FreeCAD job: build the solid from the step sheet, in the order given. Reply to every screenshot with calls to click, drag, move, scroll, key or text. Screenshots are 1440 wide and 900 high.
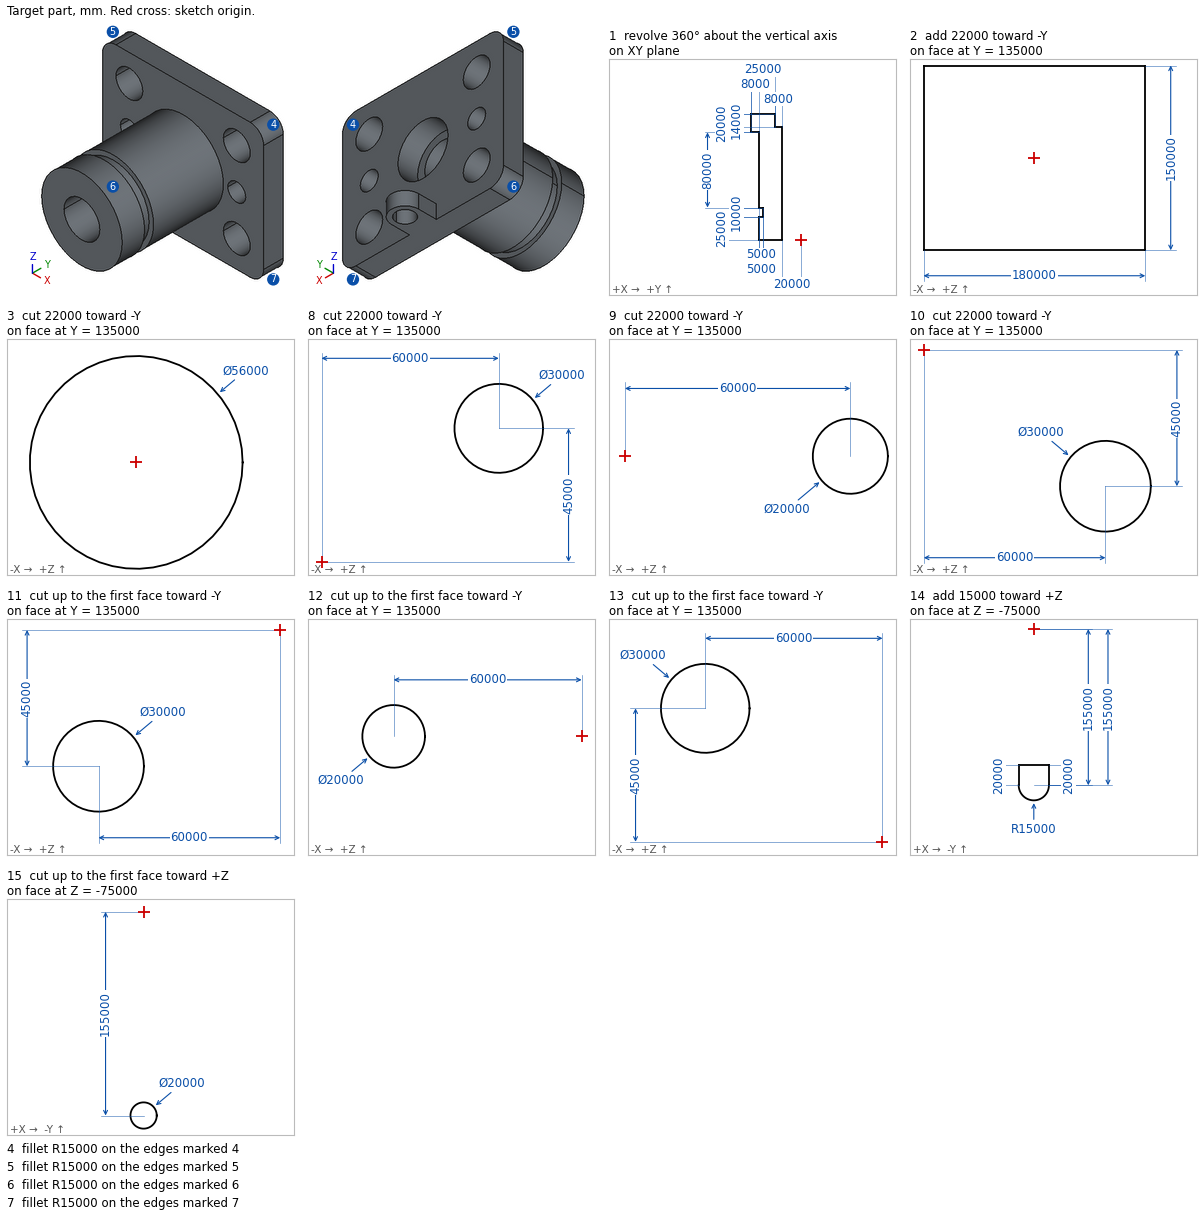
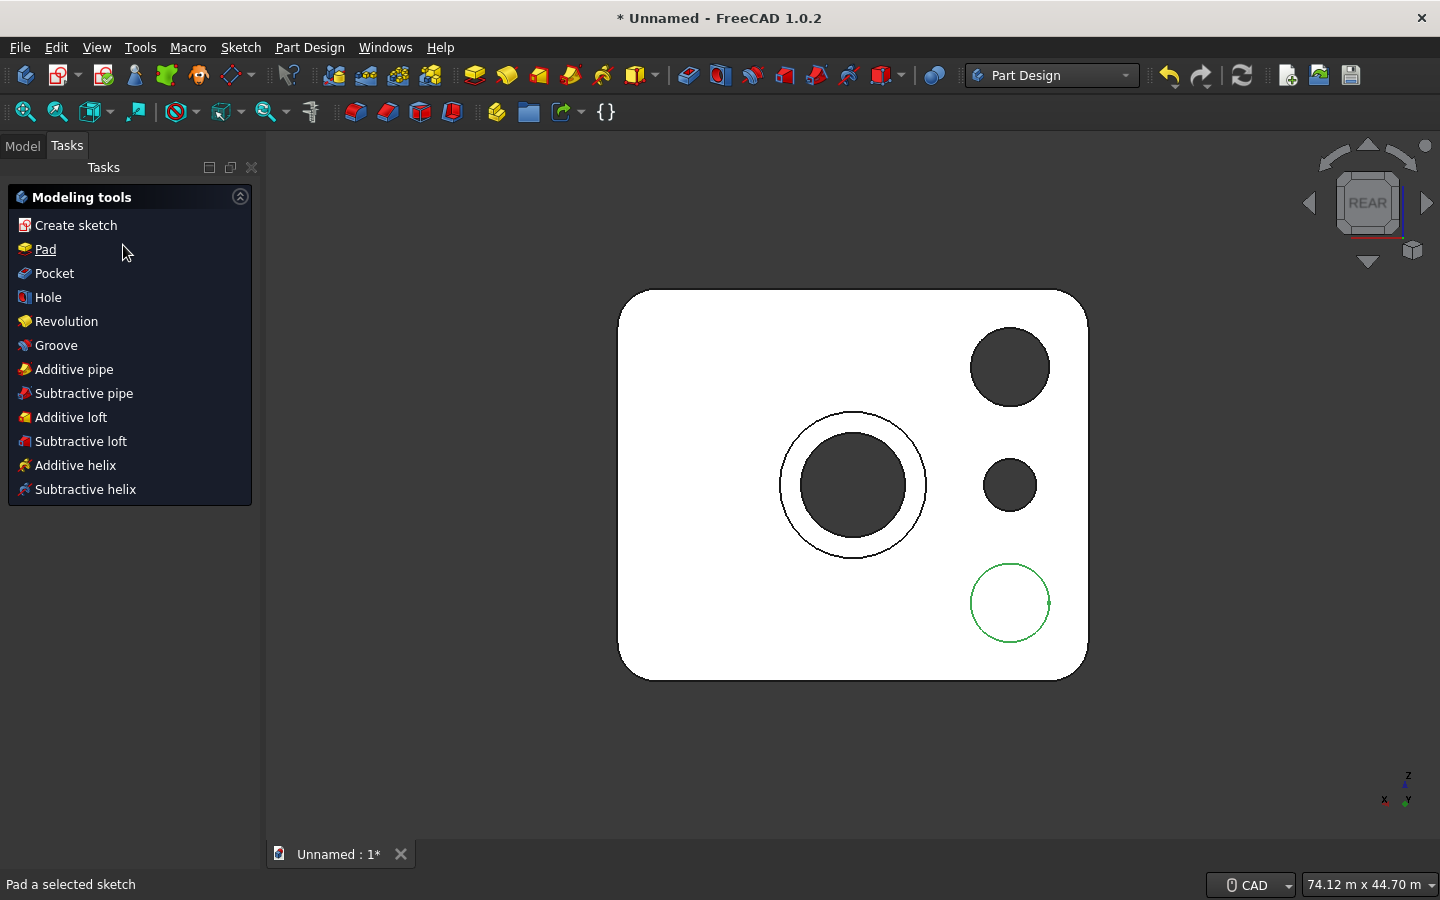
click(690, 76)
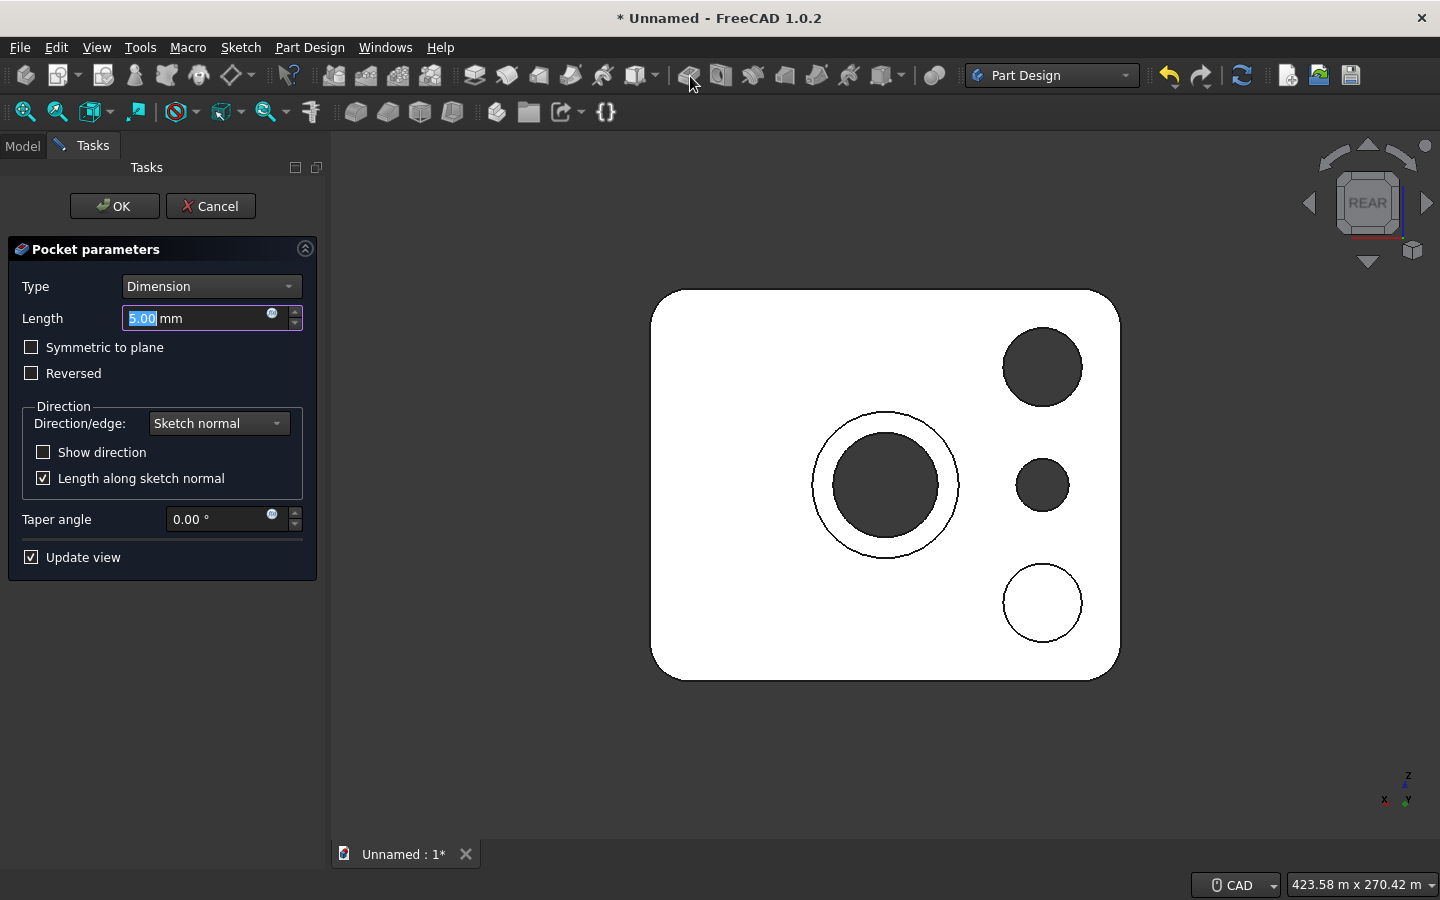
text(22000)
key(Tab)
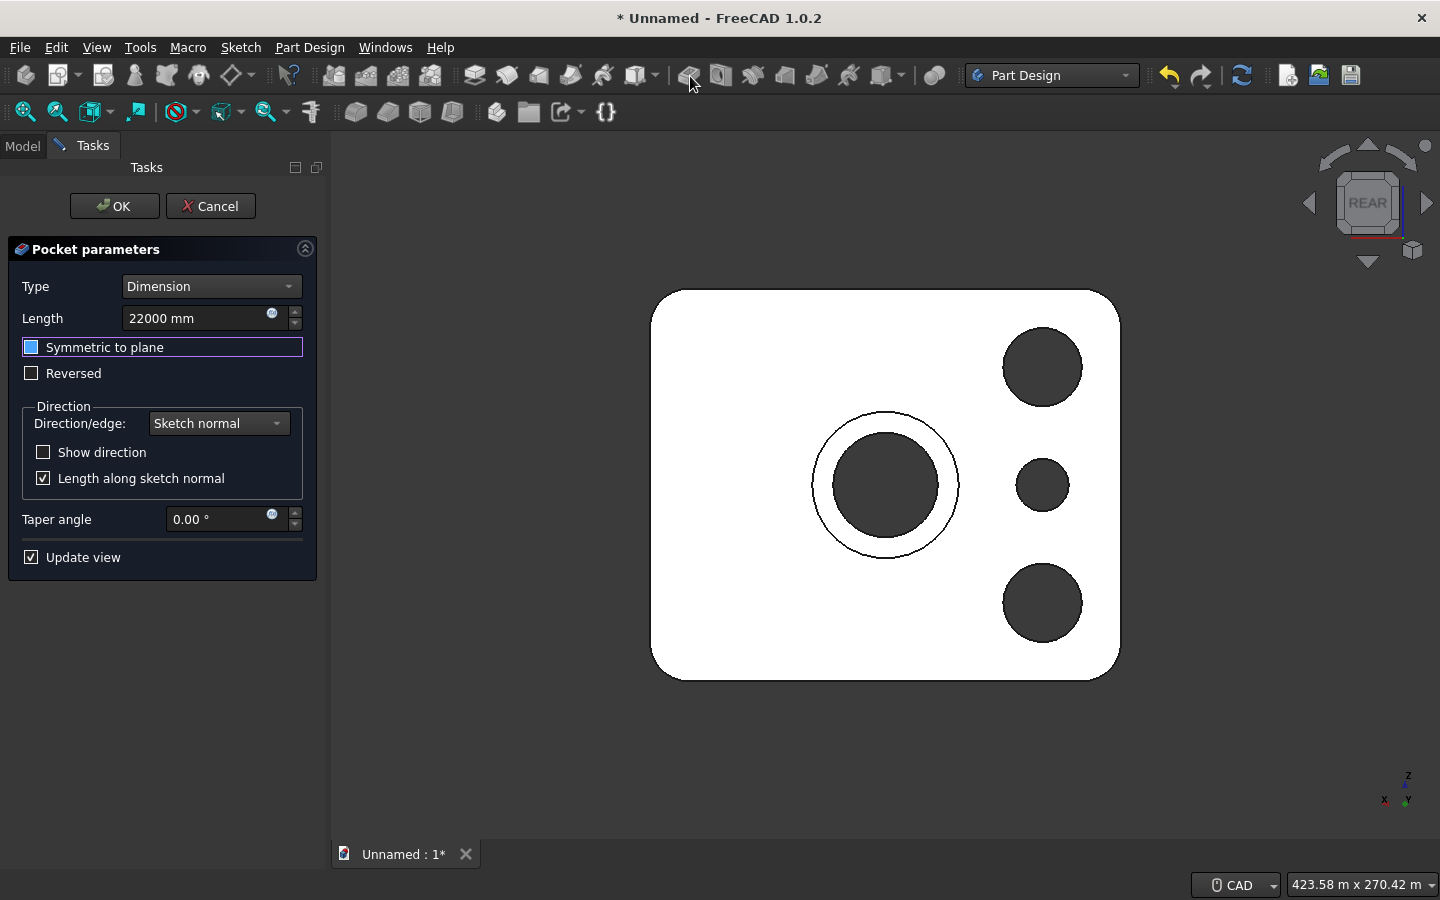
click(115, 206)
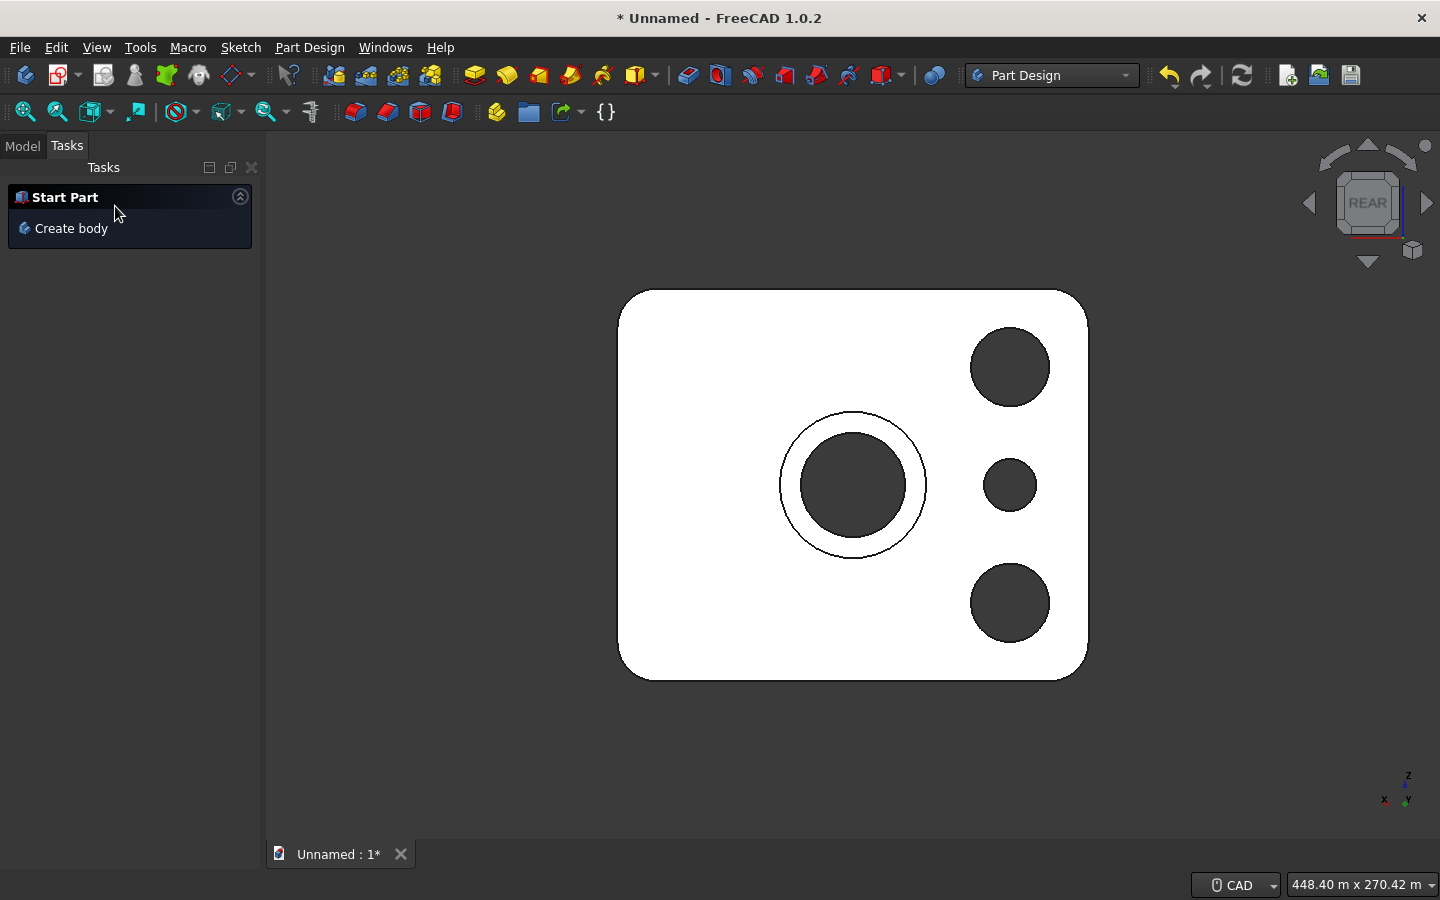
click(718, 372)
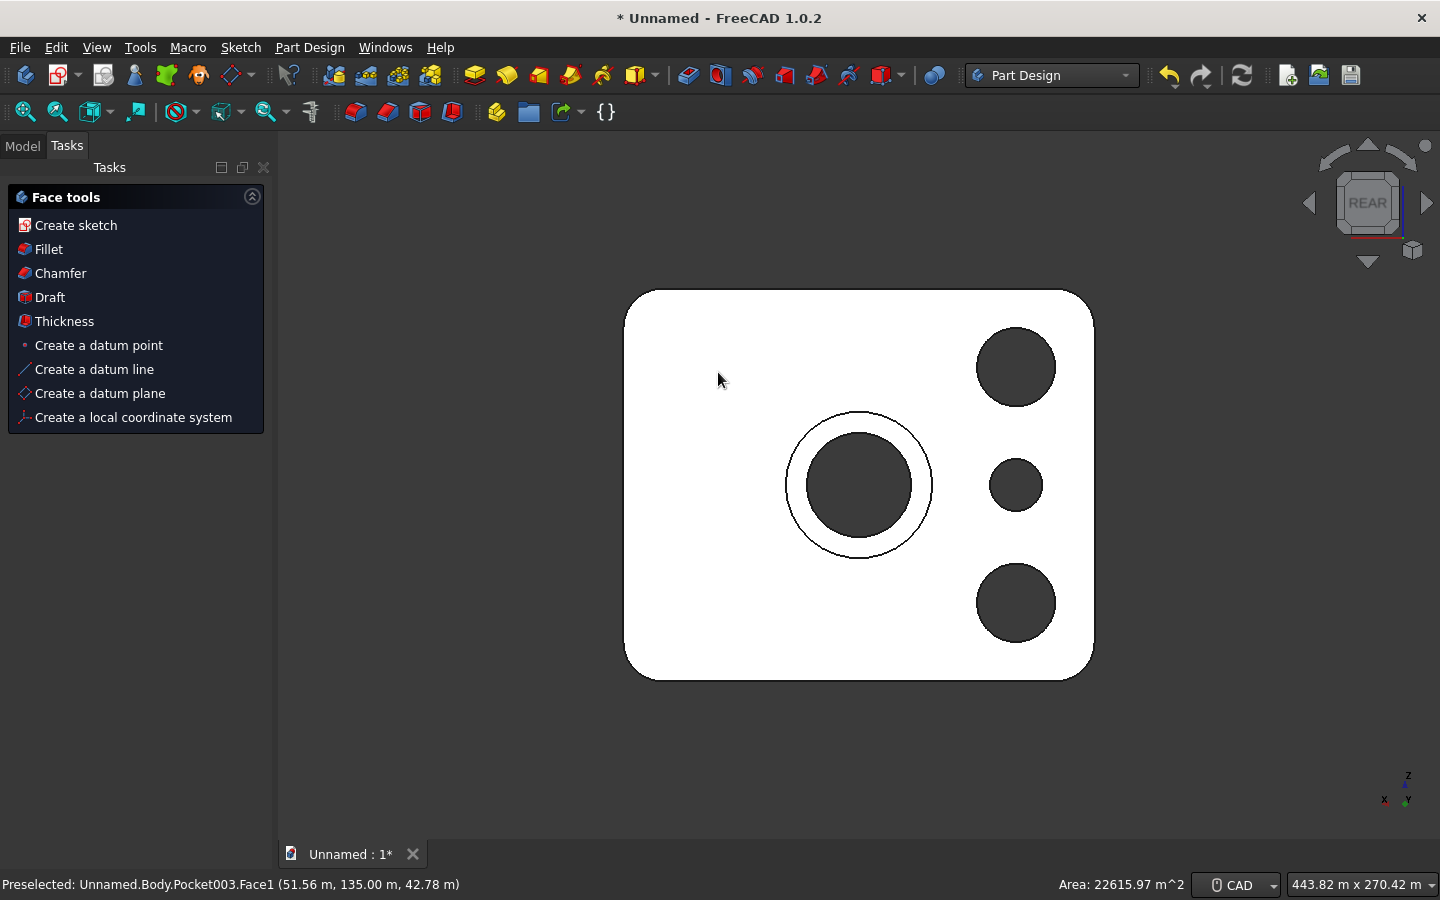
click(58, 76)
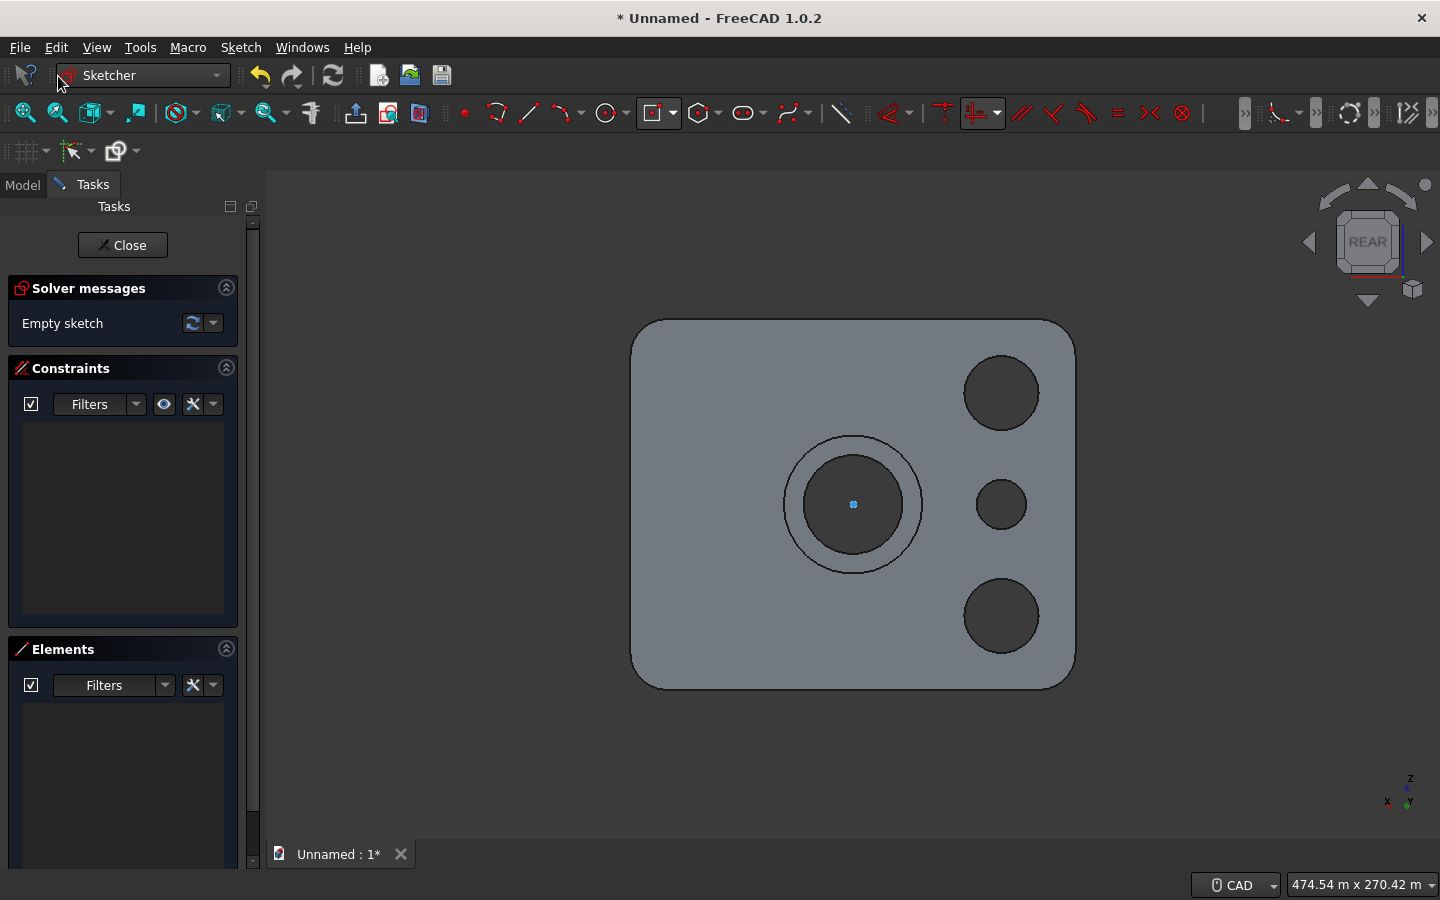
scroll(689, 638, up, 9)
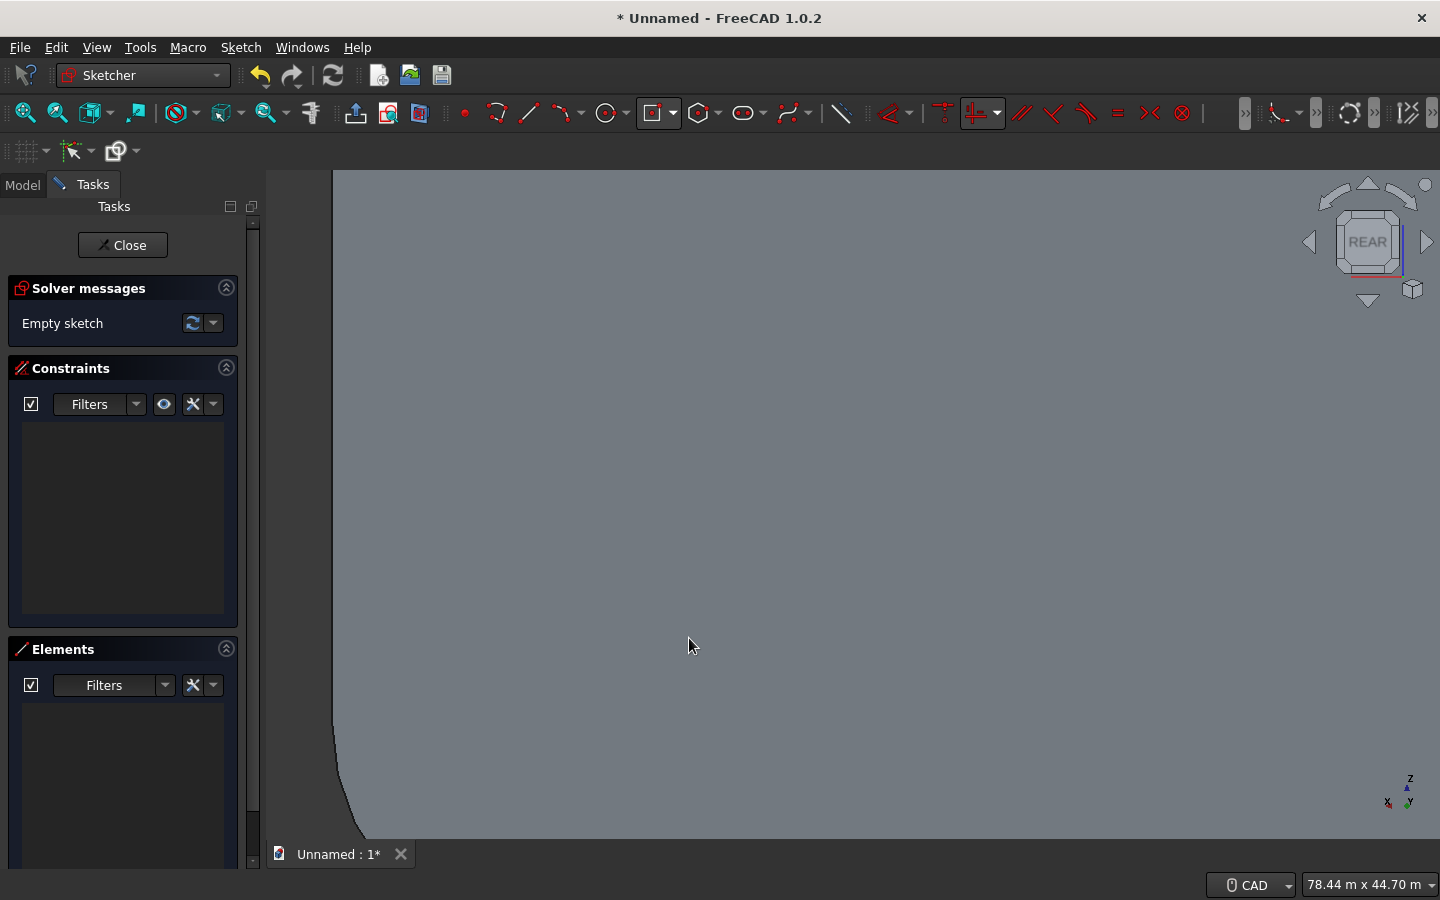
key(g)
key(c)